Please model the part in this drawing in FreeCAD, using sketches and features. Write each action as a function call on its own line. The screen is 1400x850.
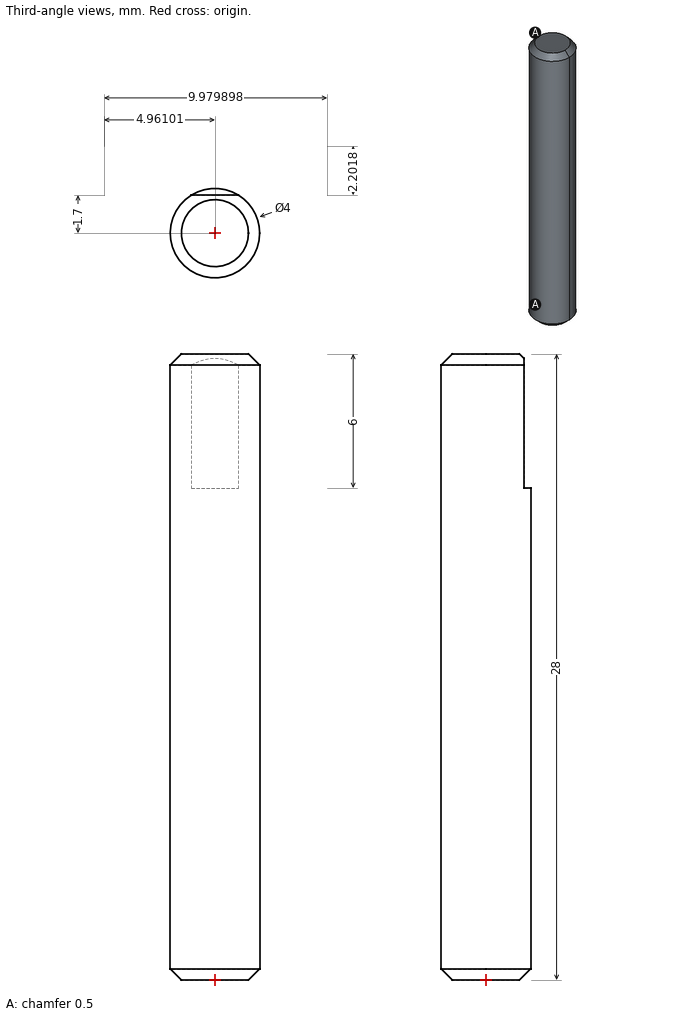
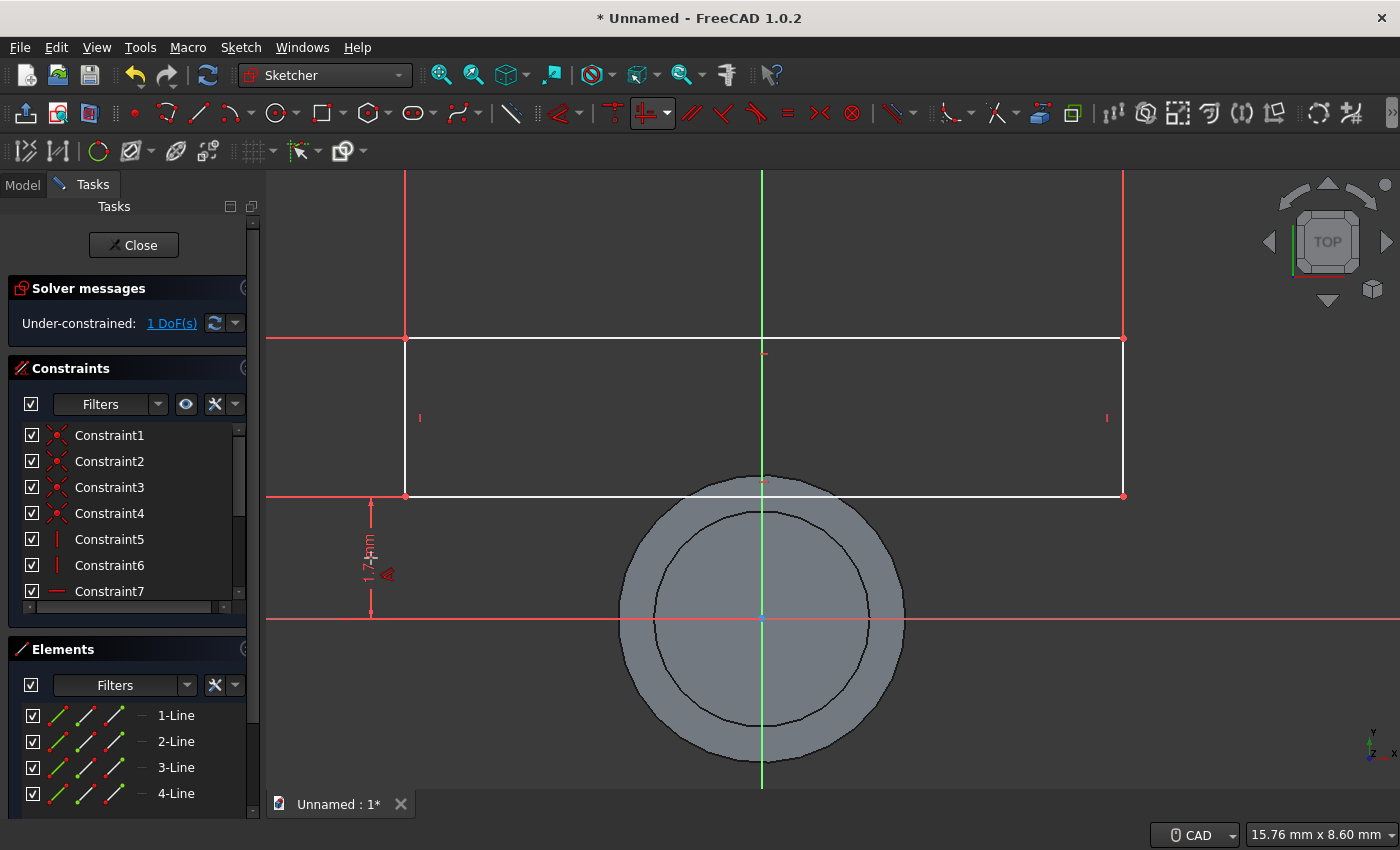
click(405, 338)
click(583, 304)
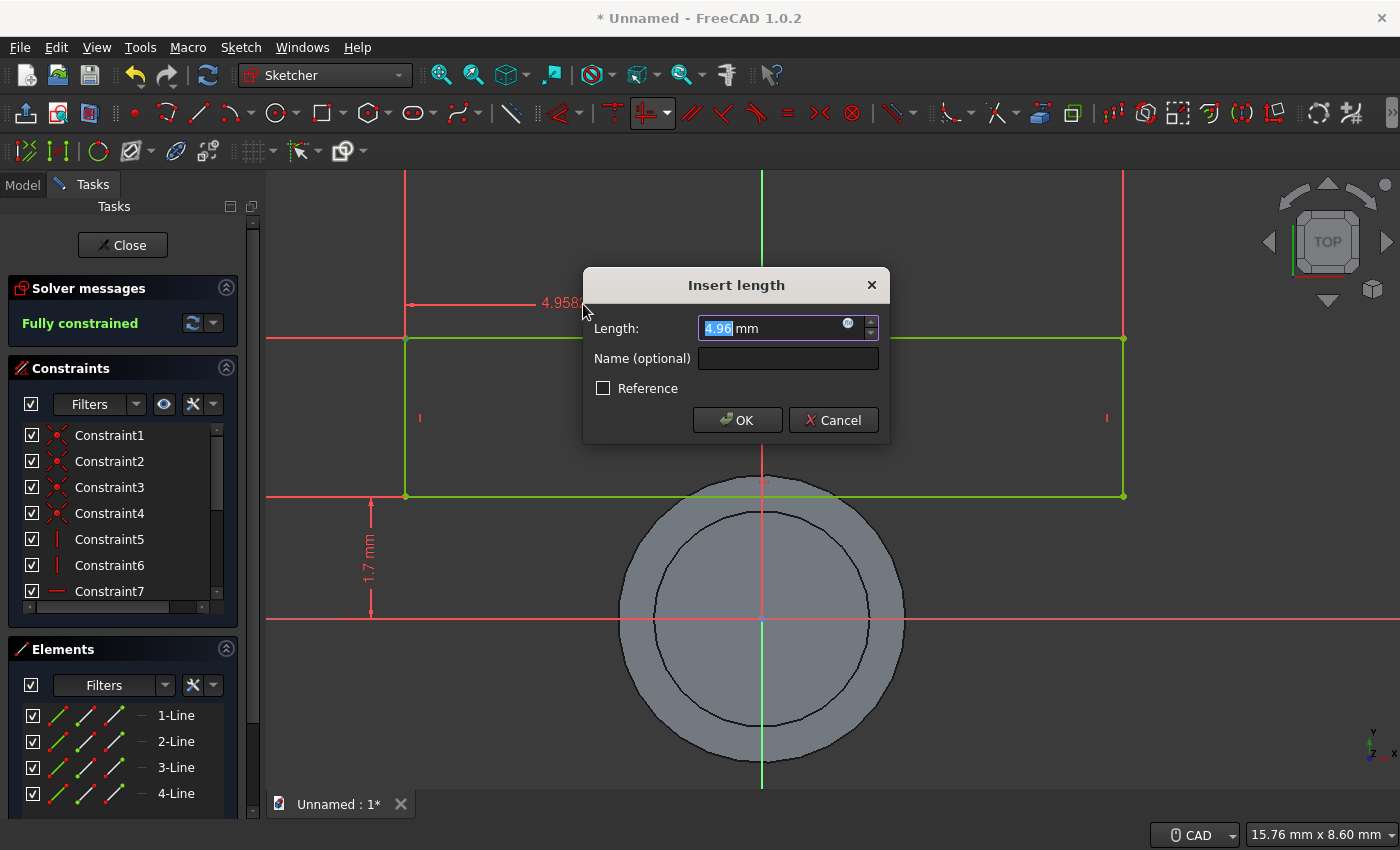
text(4.96101)
key(Return)
key(Escape)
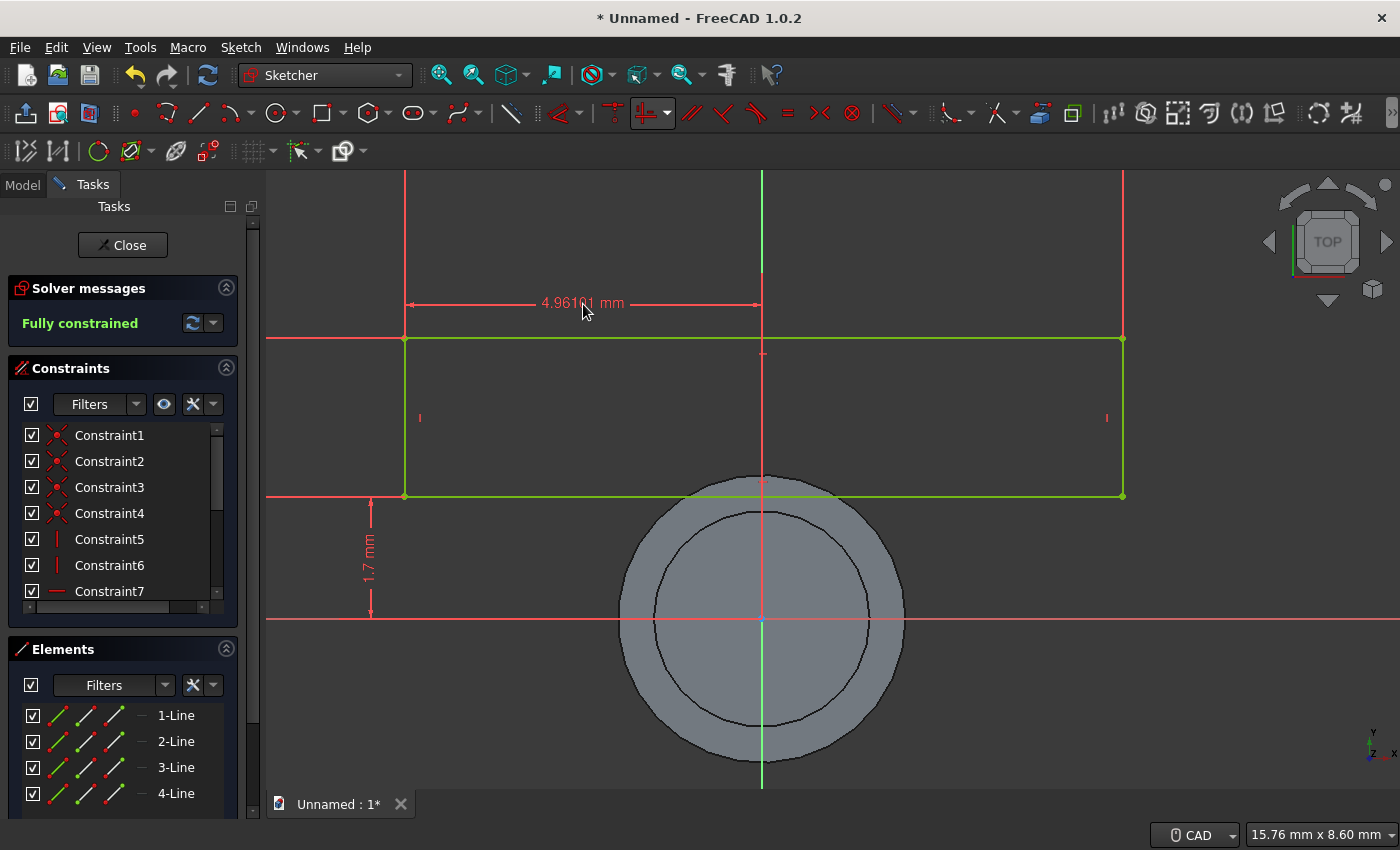
click(123, 245)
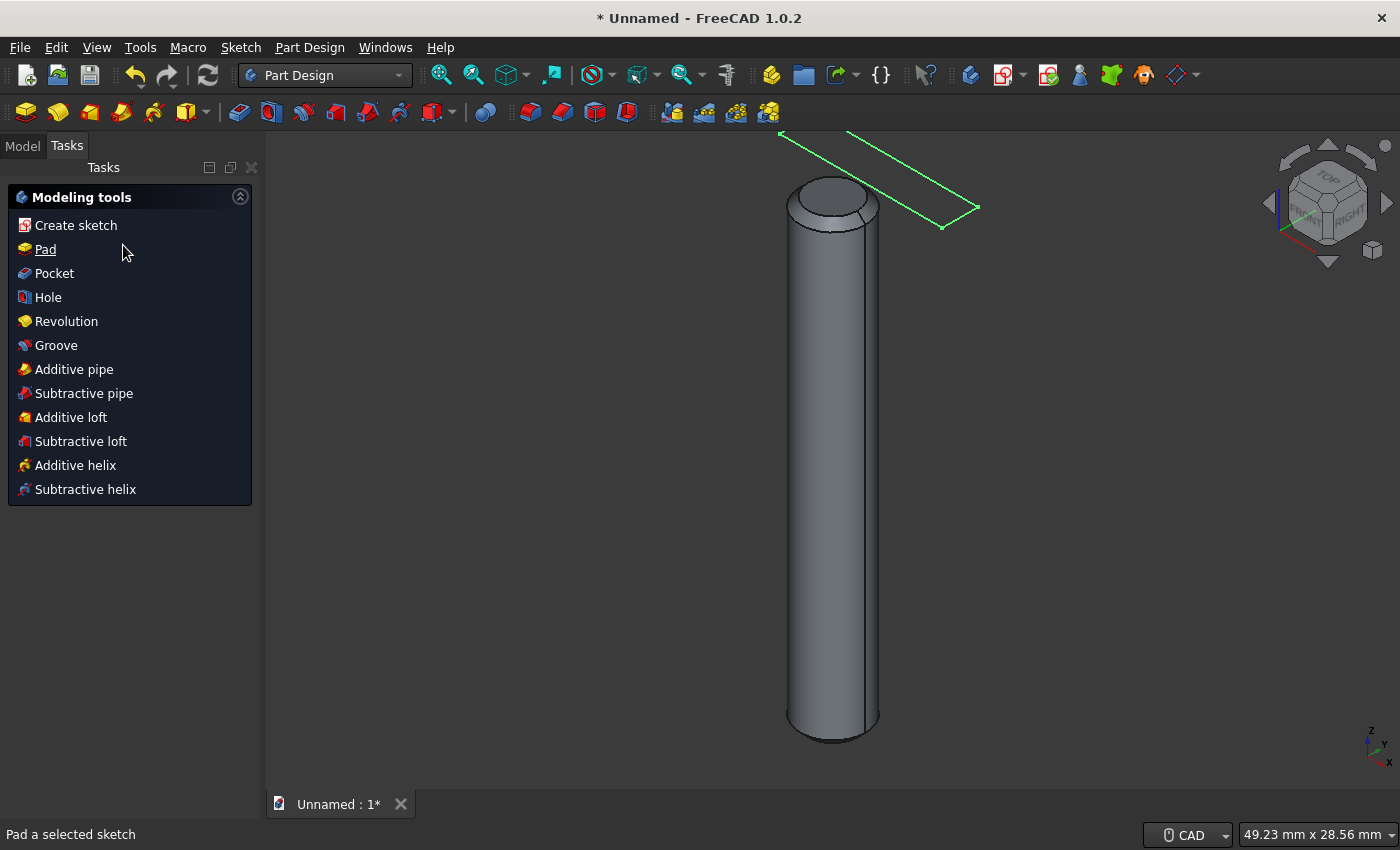
click(240, 112)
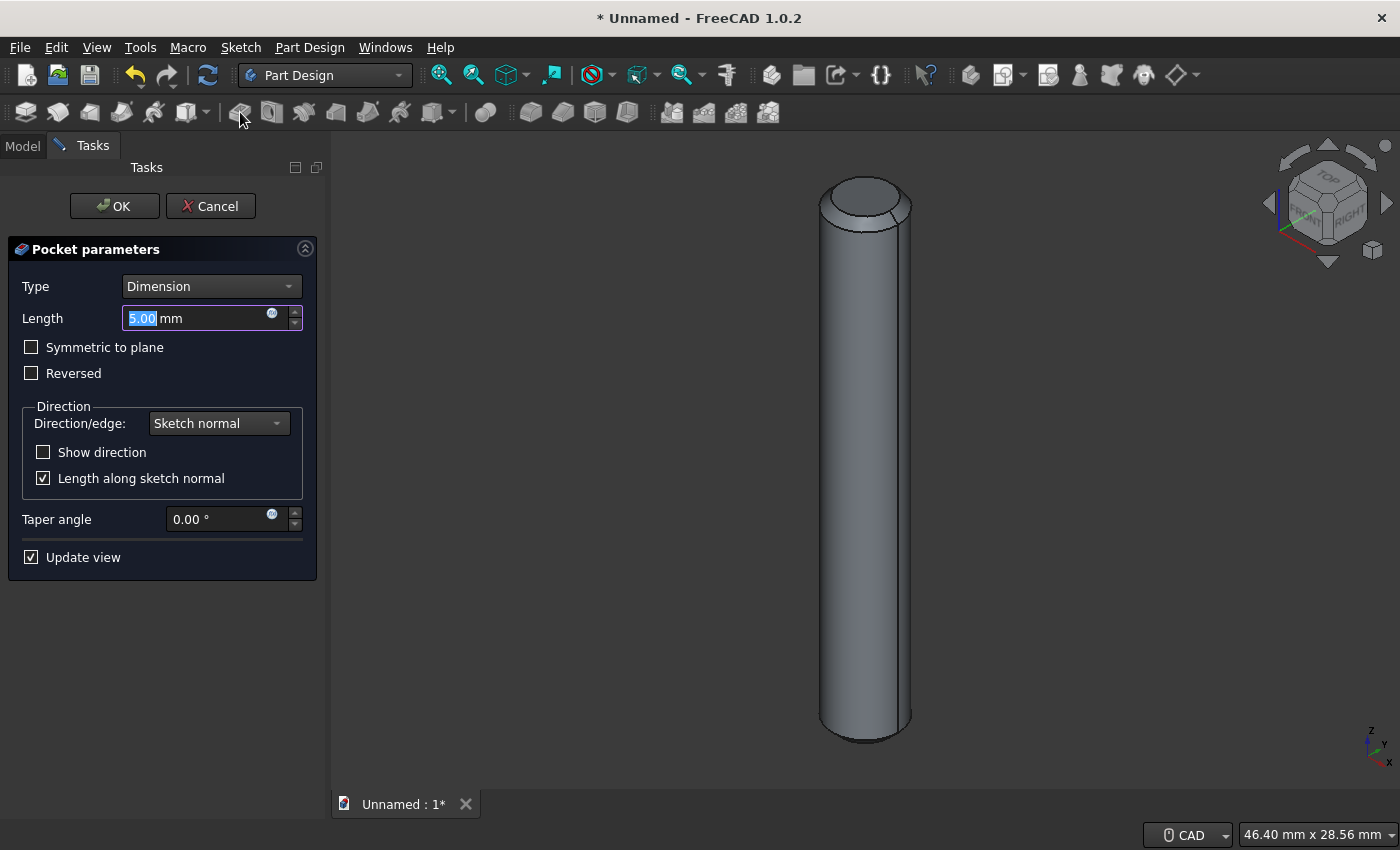
text(6)
key(Tab)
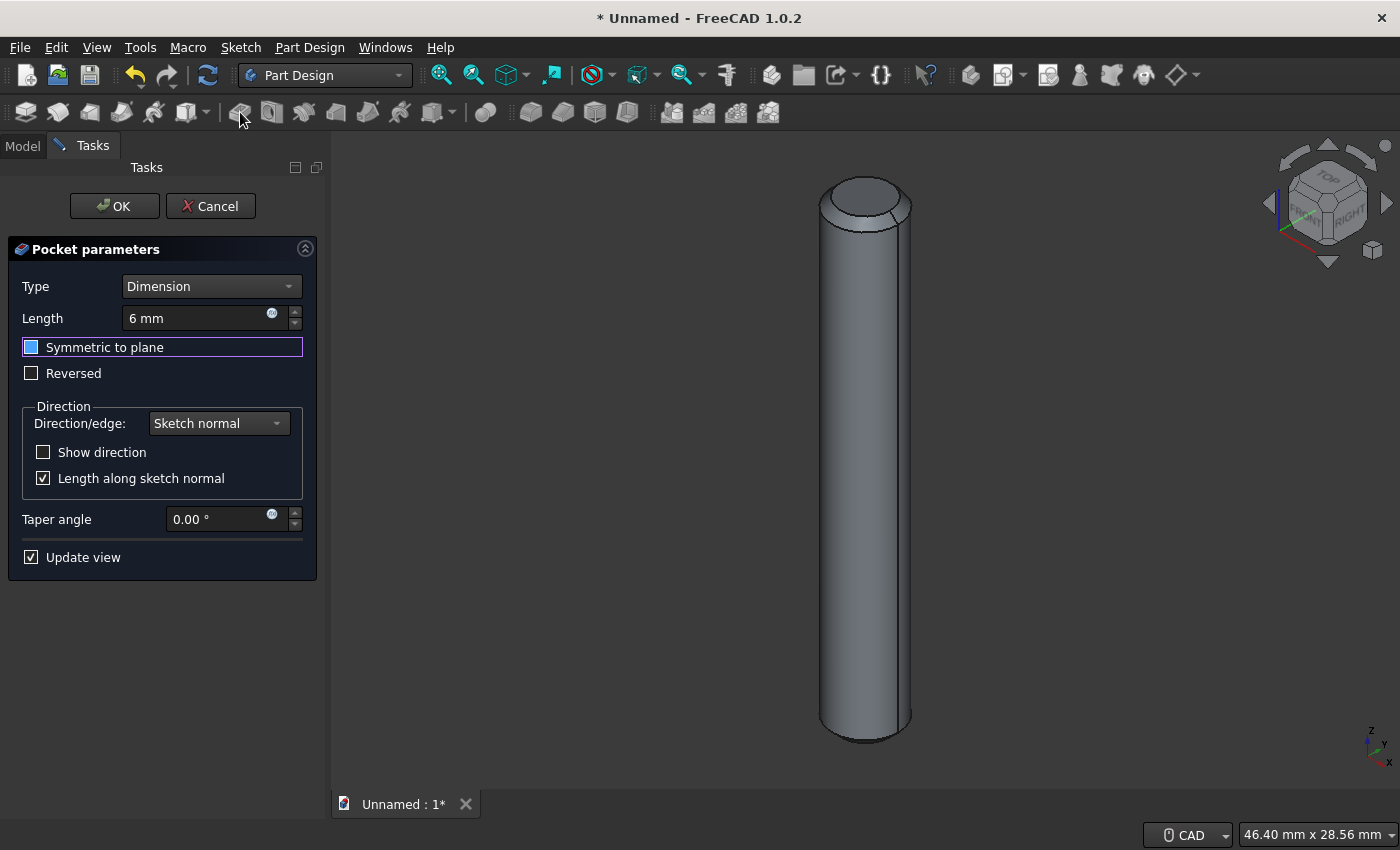
click(115, 206)